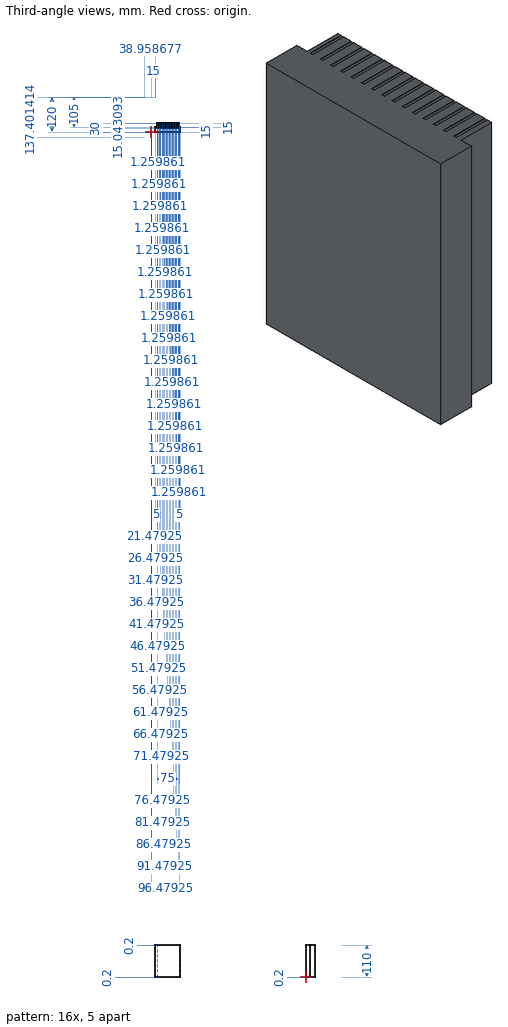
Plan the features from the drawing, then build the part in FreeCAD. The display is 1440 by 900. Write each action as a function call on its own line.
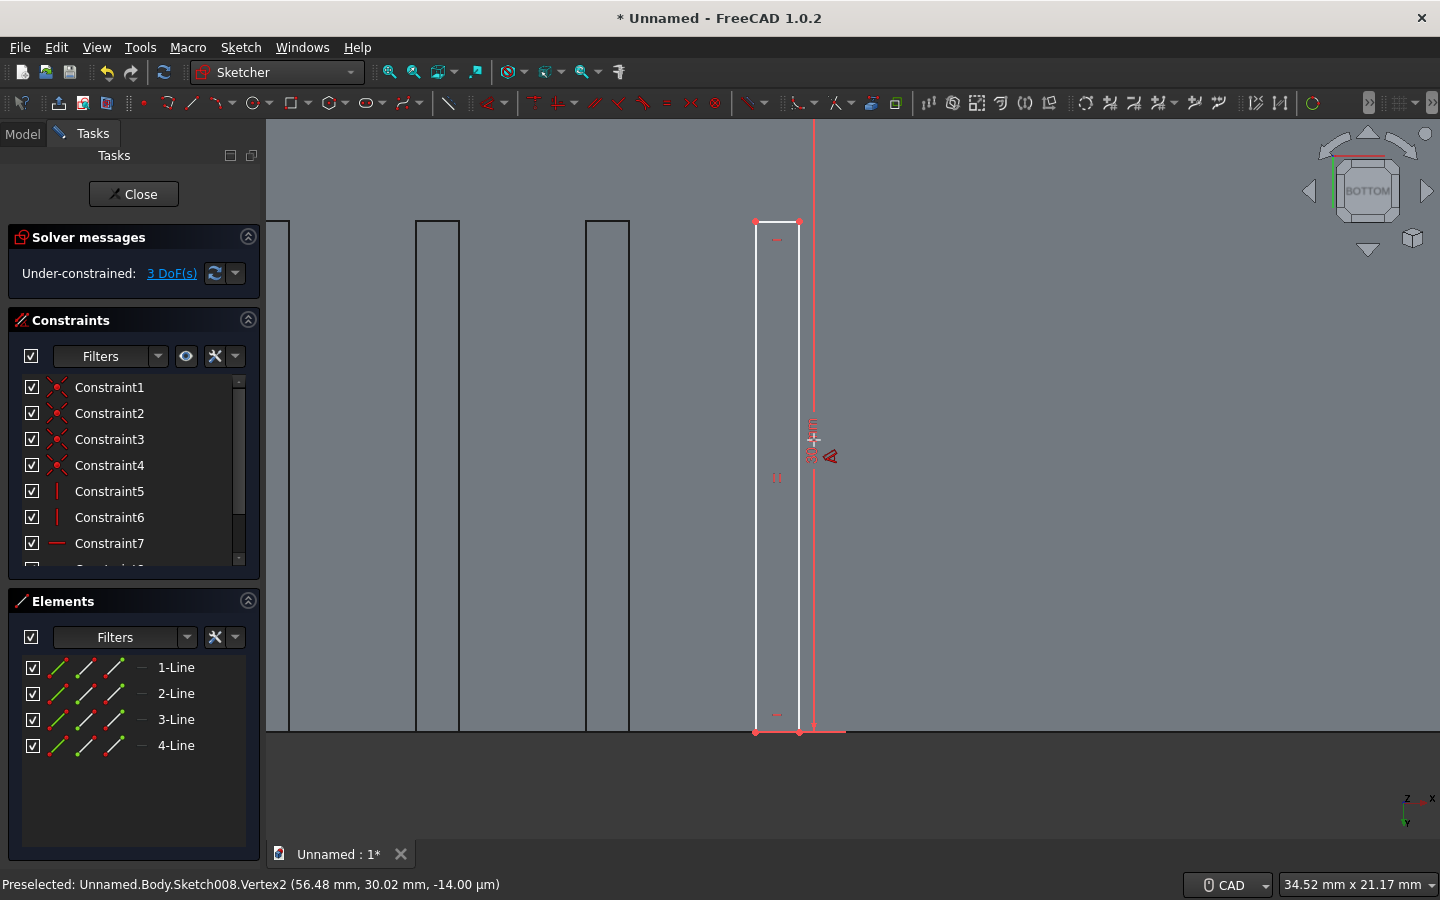
click(769, 732)
click(777, 766)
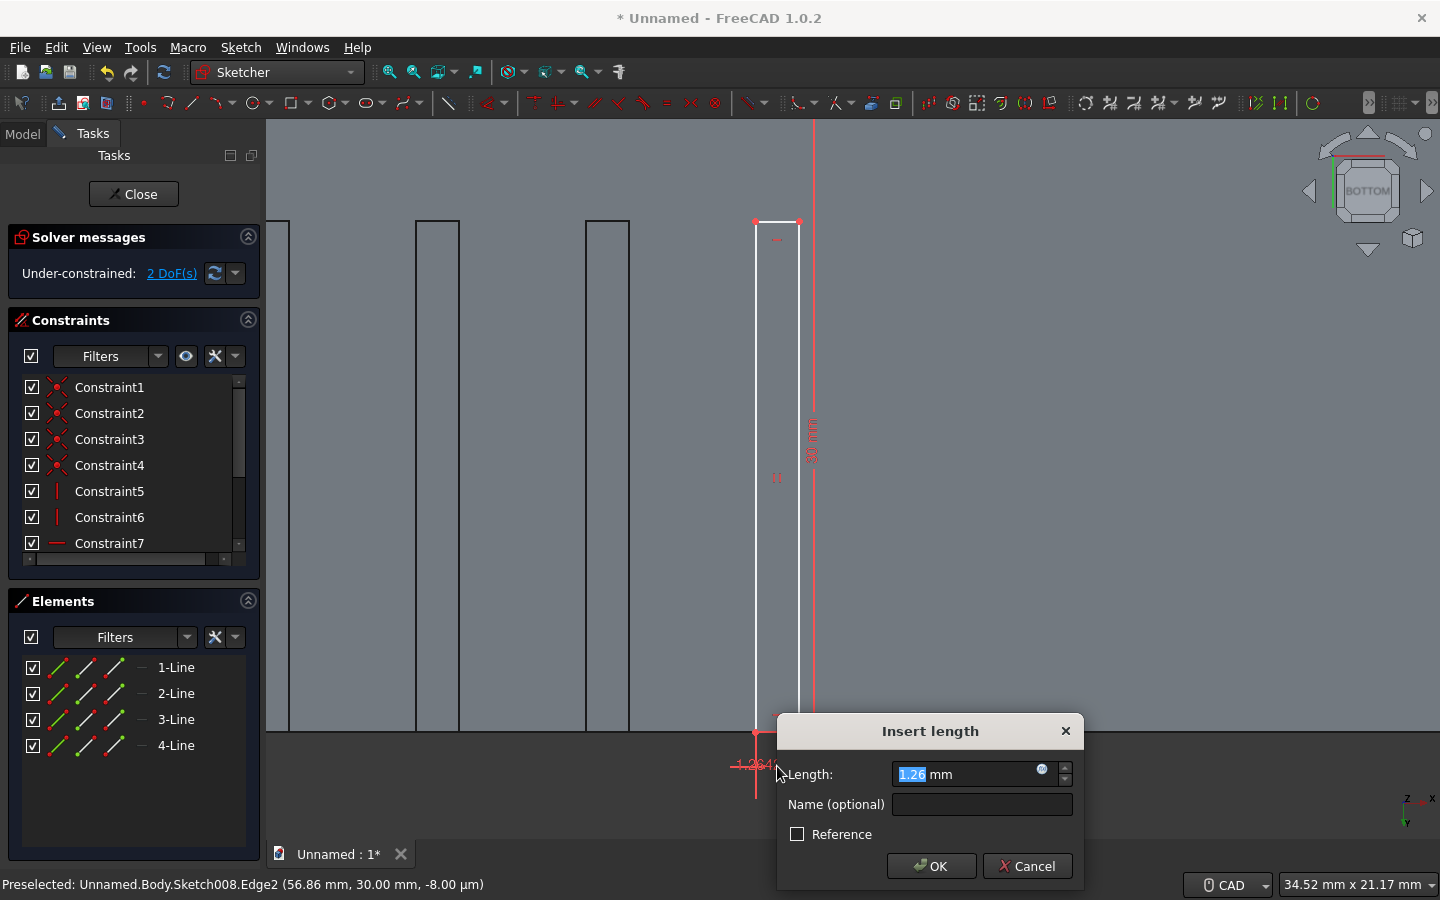
text(1.259861)
key(Return)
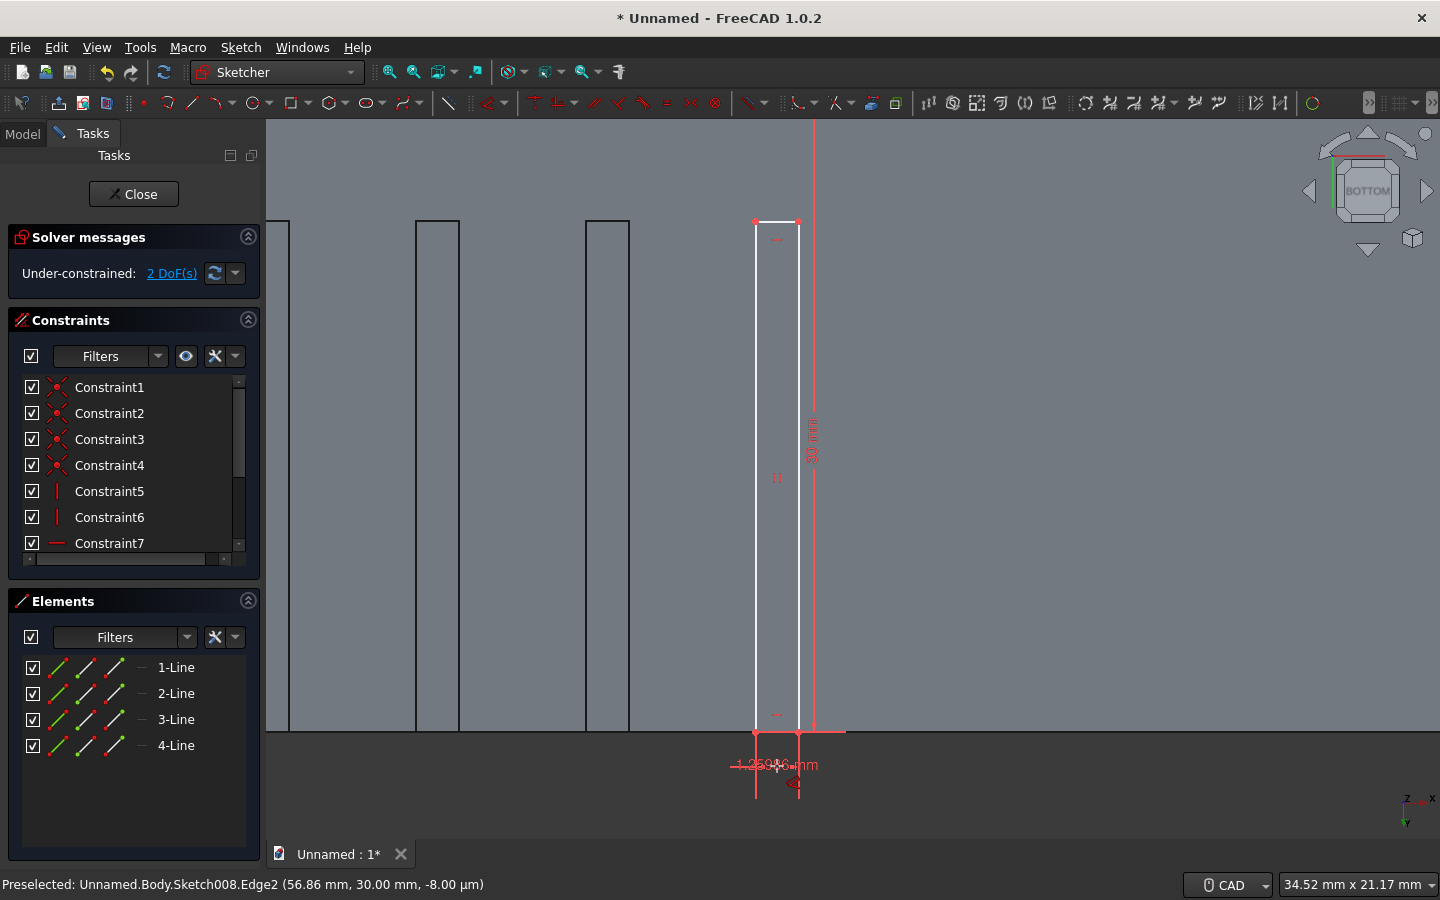
click(756, 375)
click(722, 477)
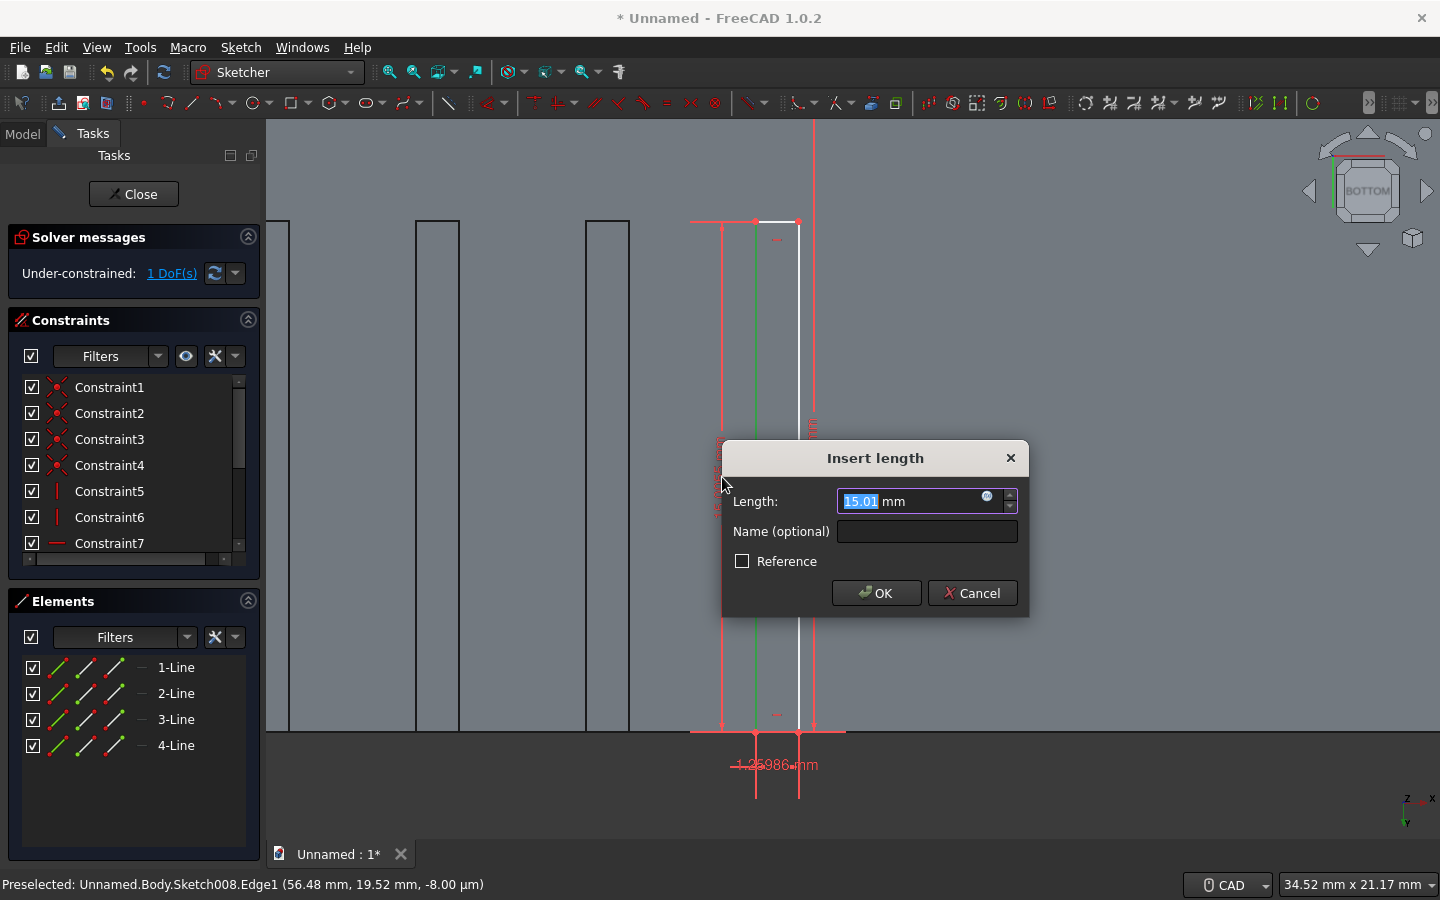
text(15.043093)
key(Return)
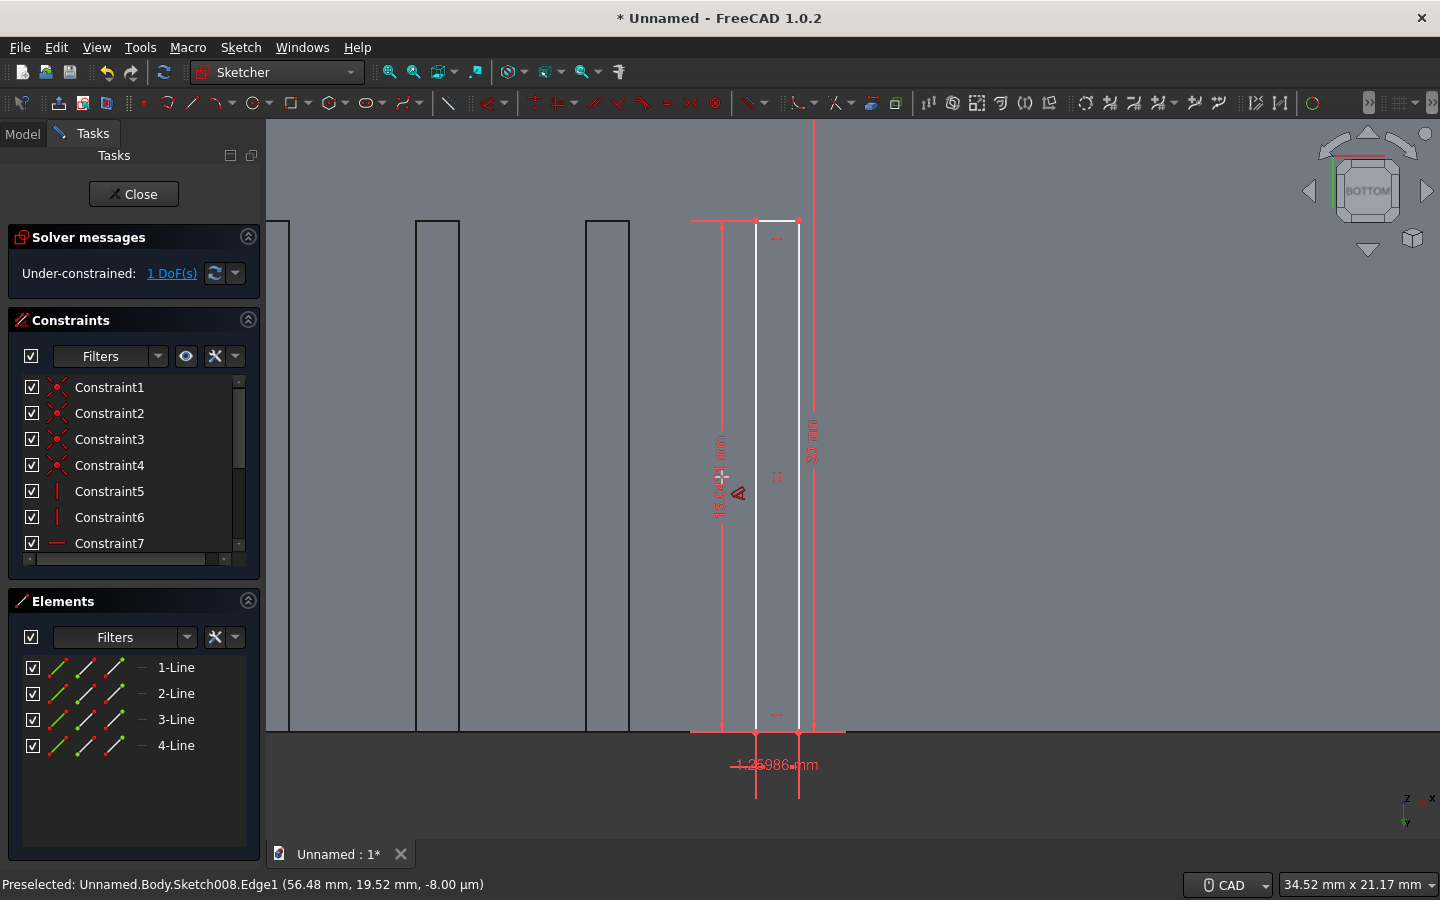
click(756, 221)
click(525, 255)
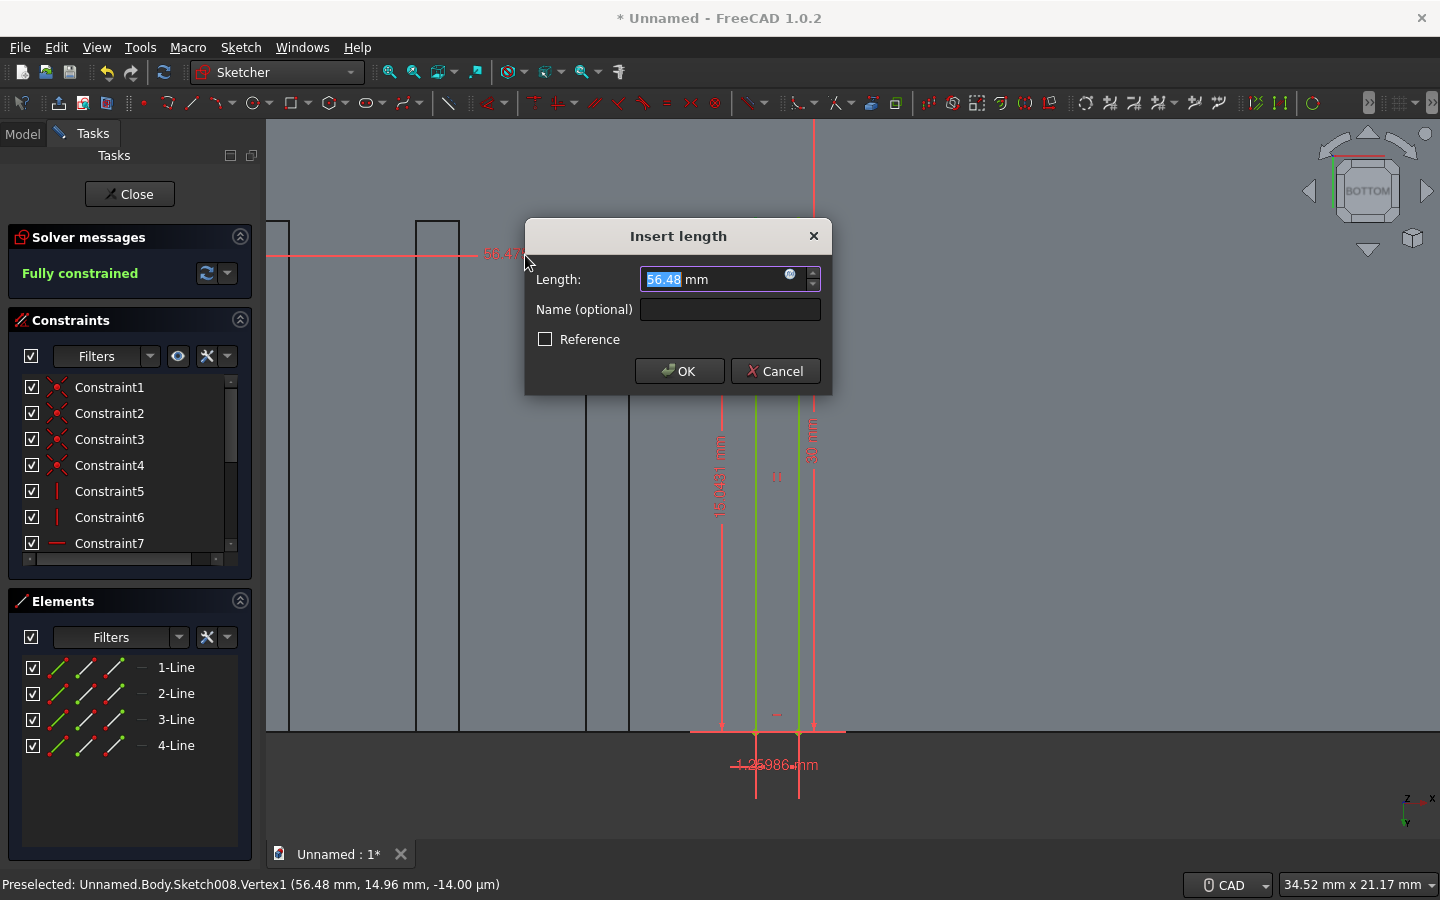
text(56.47925)
key(Return)
key(Escape)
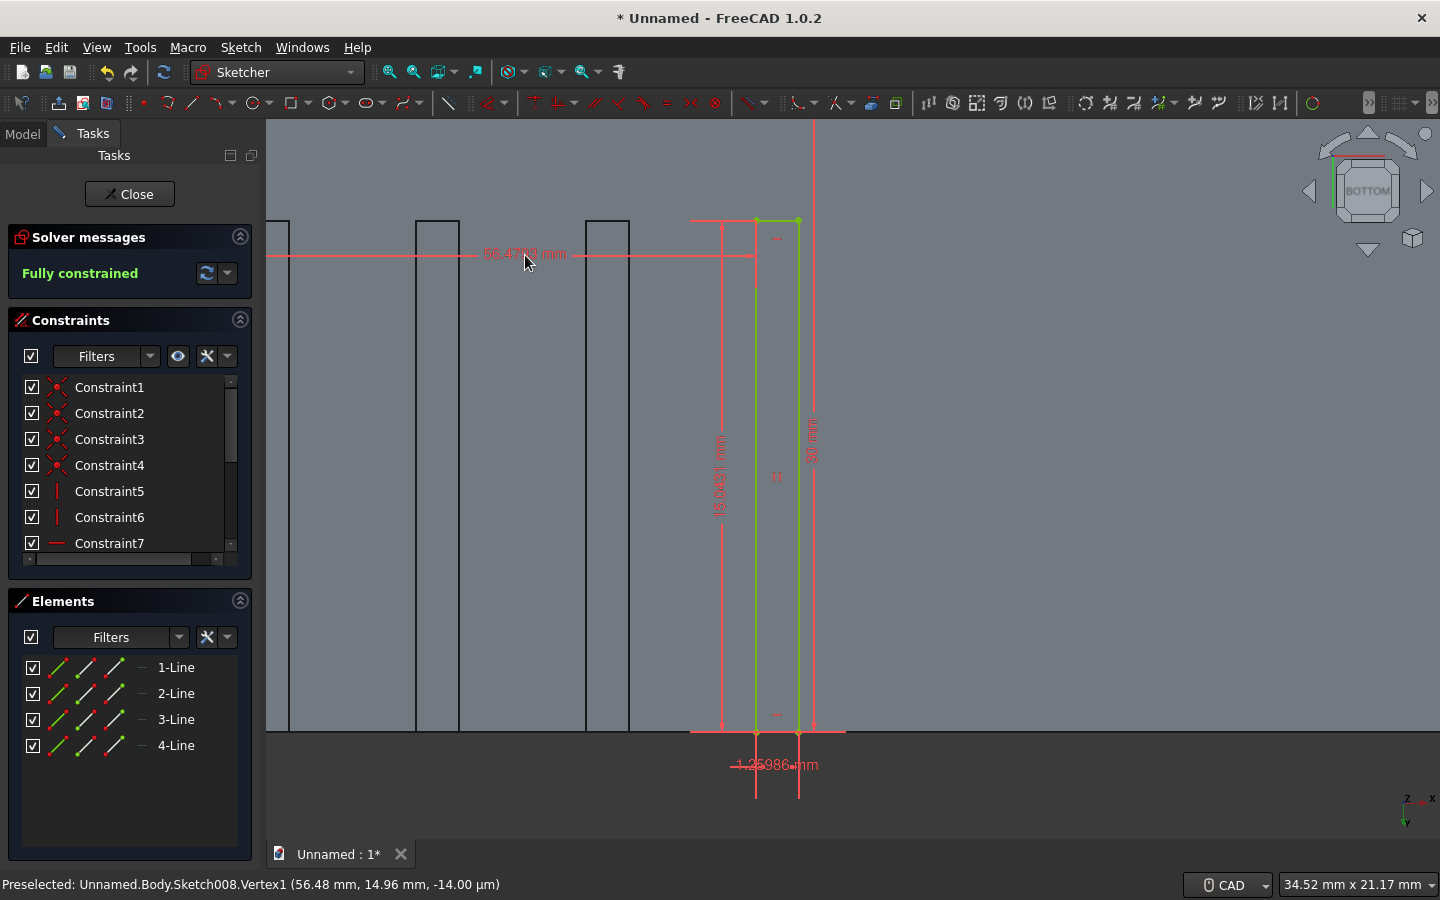
click(130, 194)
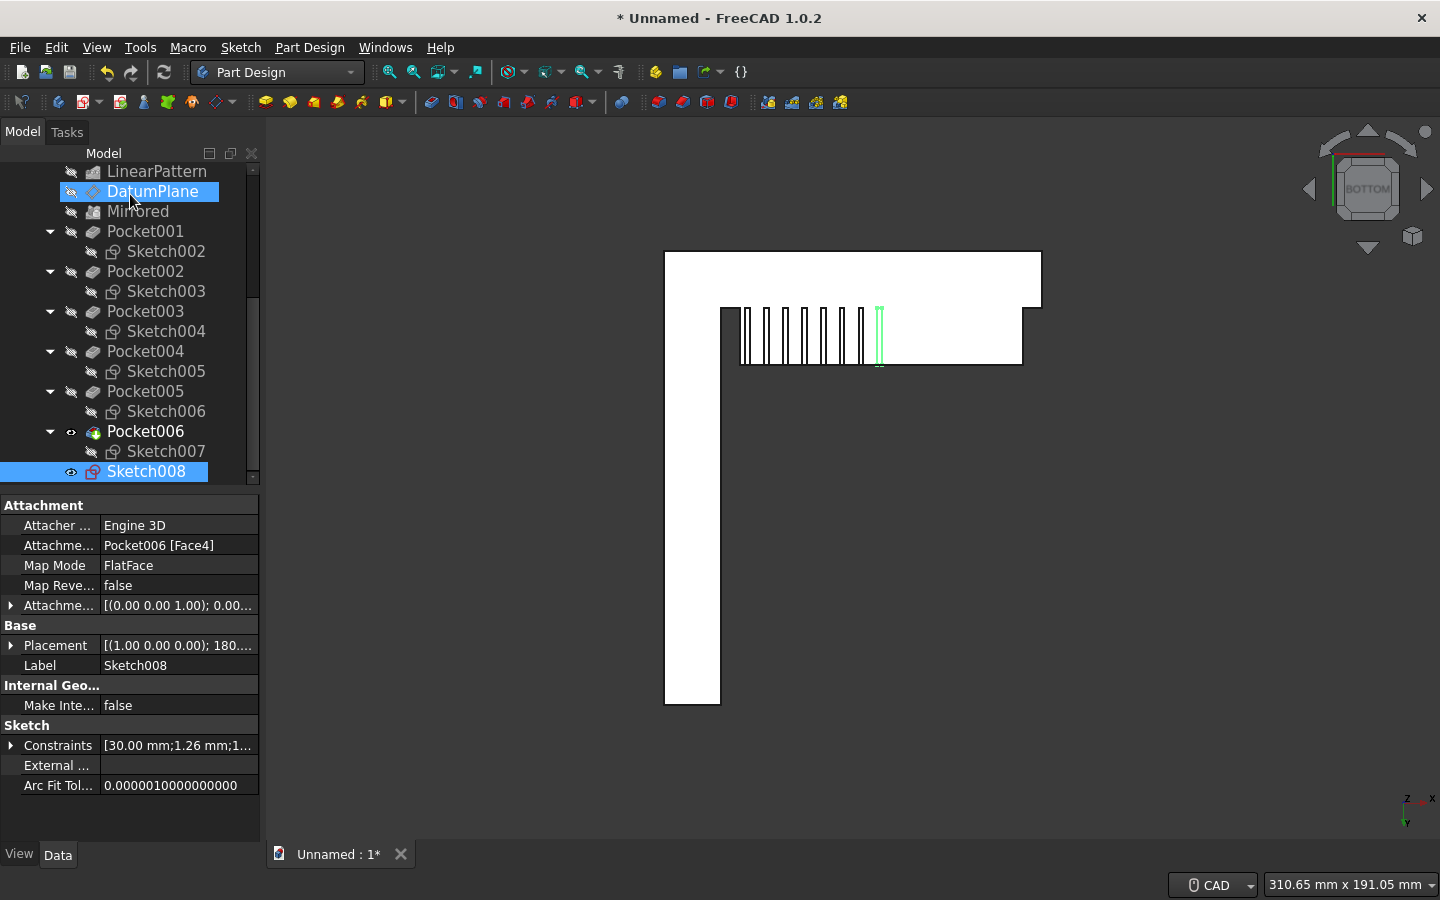
click(432, 102)